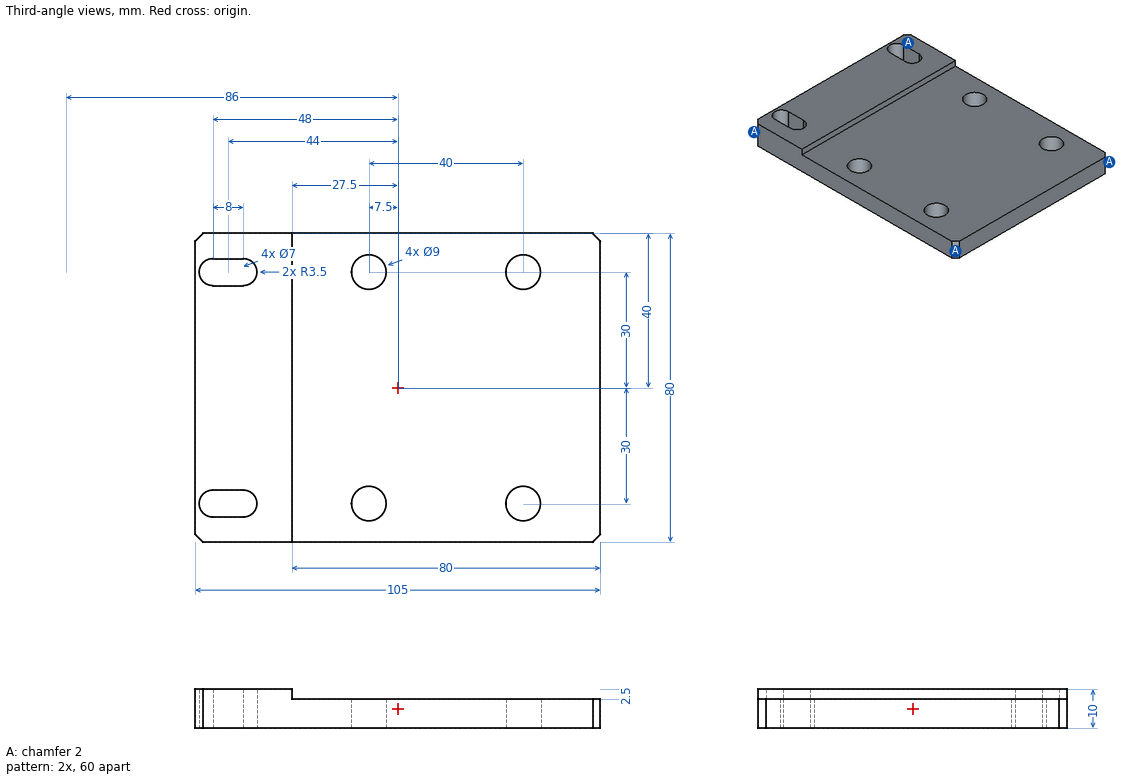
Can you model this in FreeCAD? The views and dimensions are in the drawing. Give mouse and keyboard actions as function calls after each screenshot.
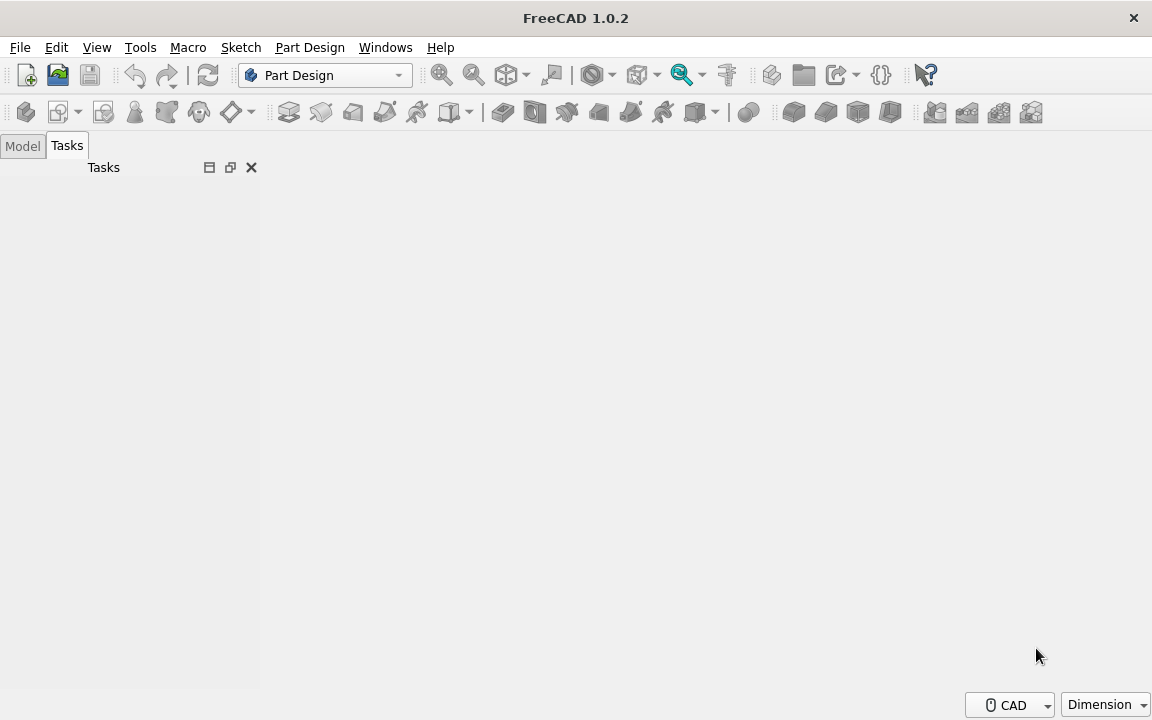
click(26, 76)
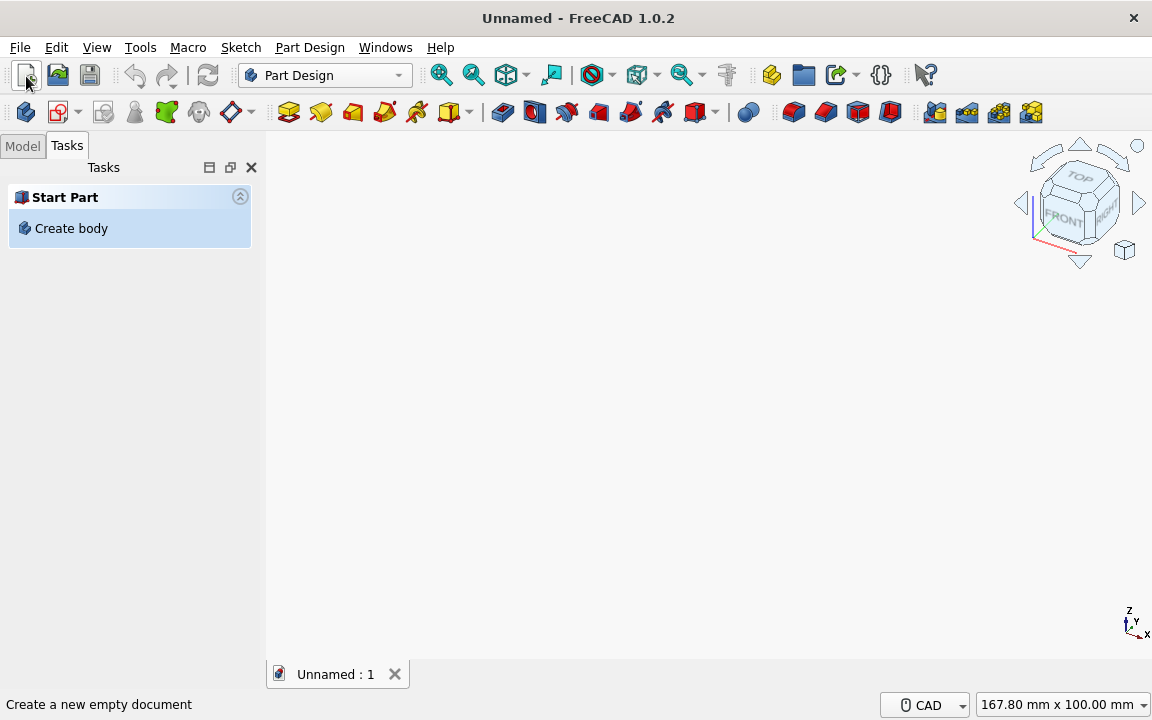
click(58, 112)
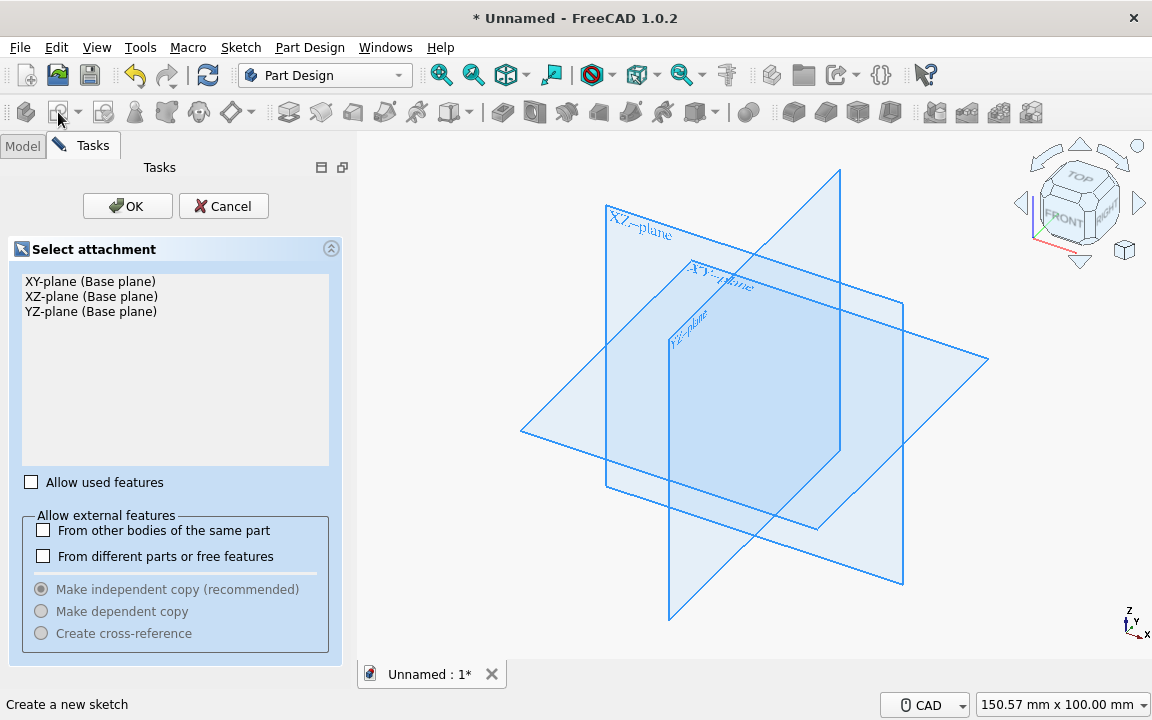
click(82, 282)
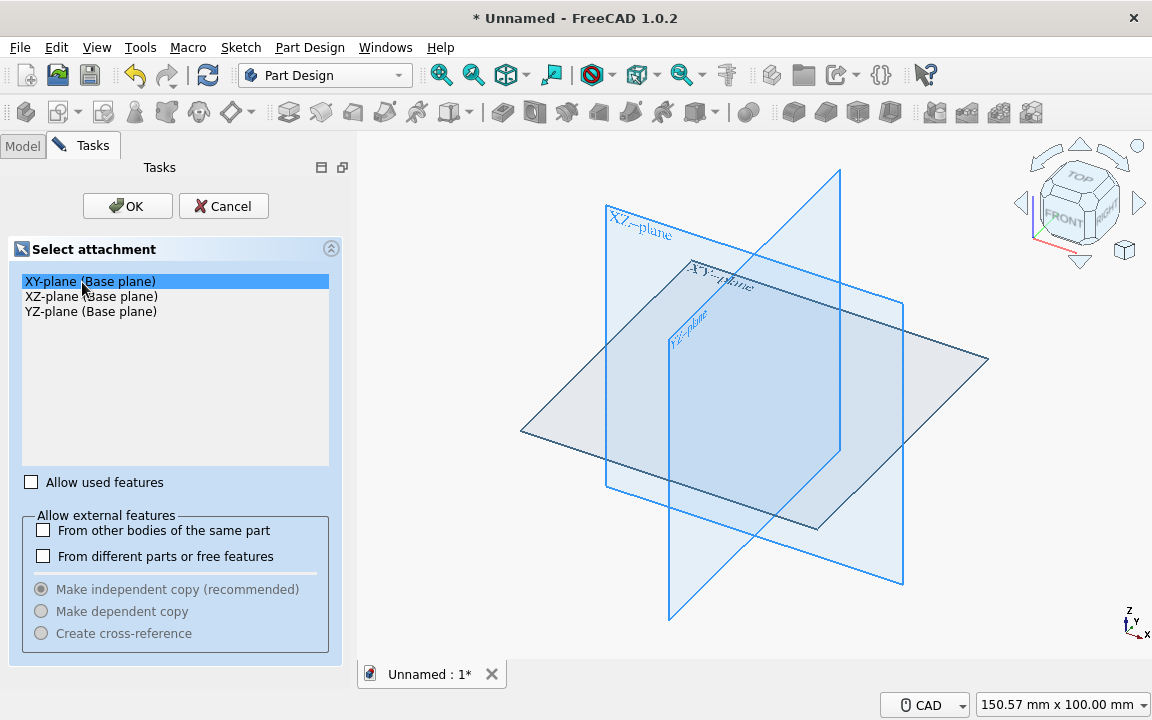
click(128, 206)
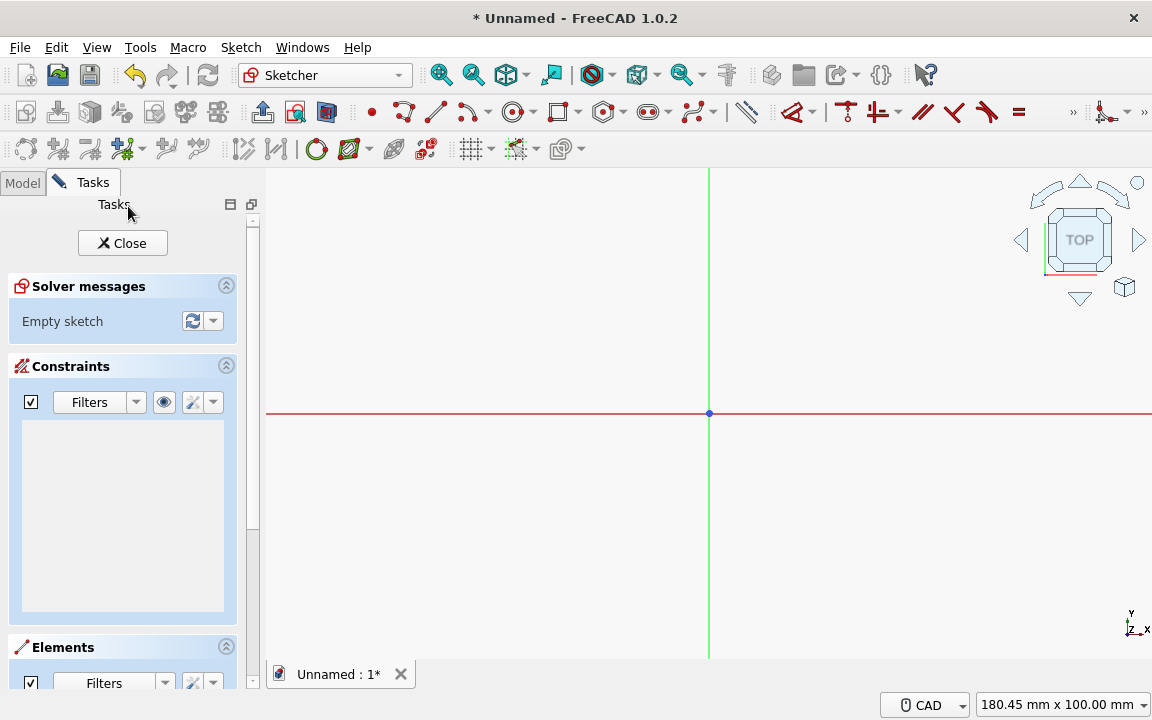
scroll(331, 413, down, 1)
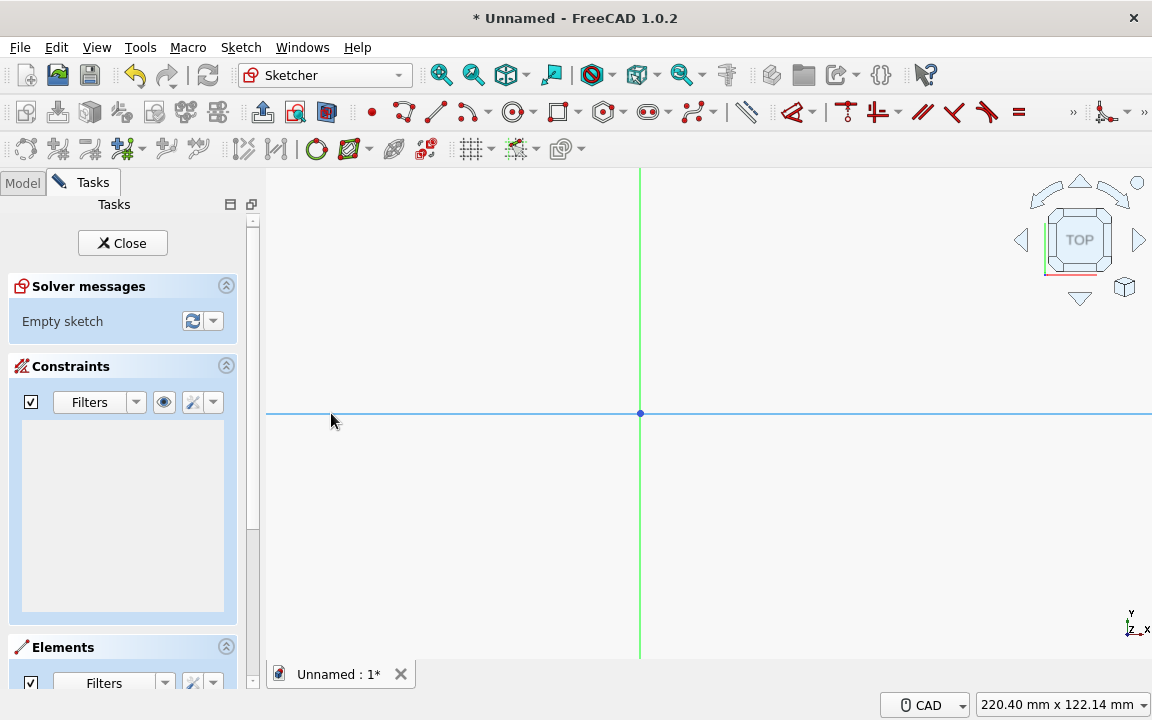
key(g)
key(v)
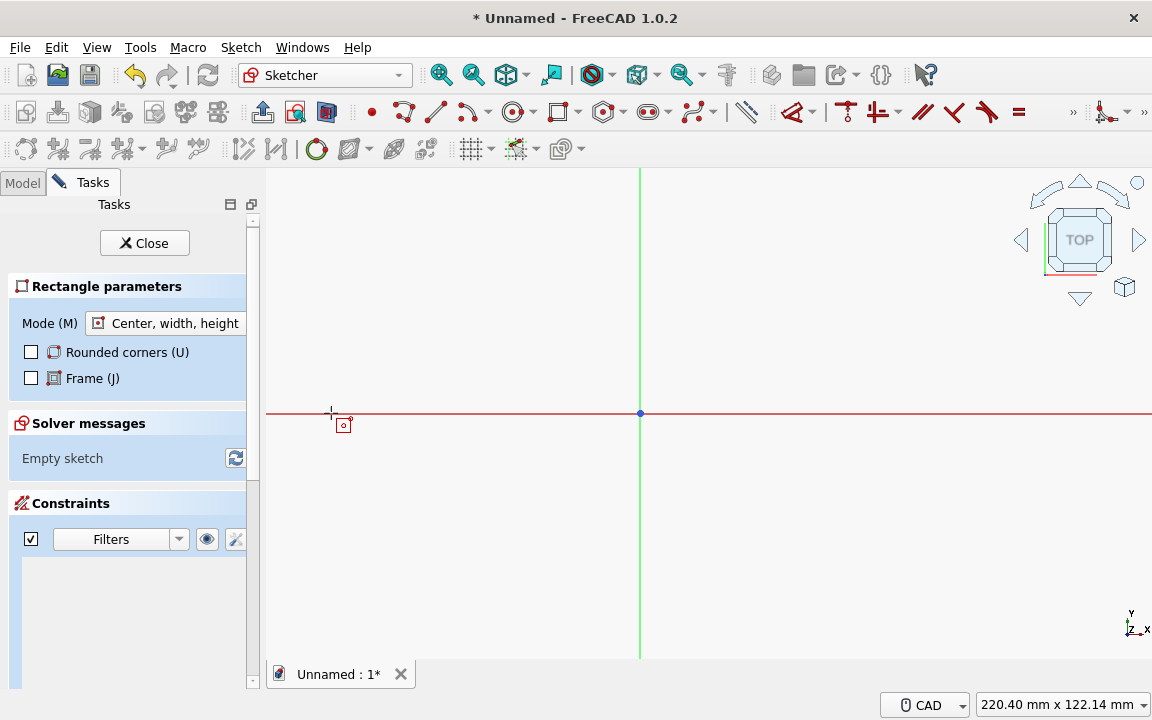
click(640, 414)
click(852, 253)
key(Escape)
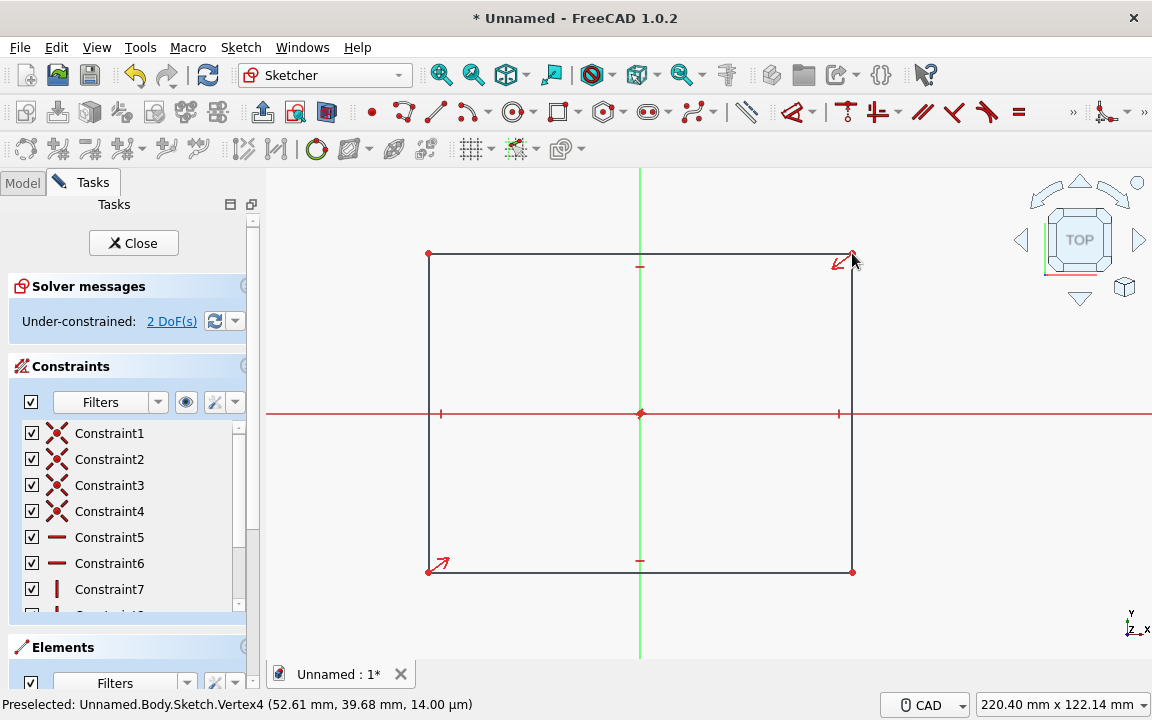
click(852, 477)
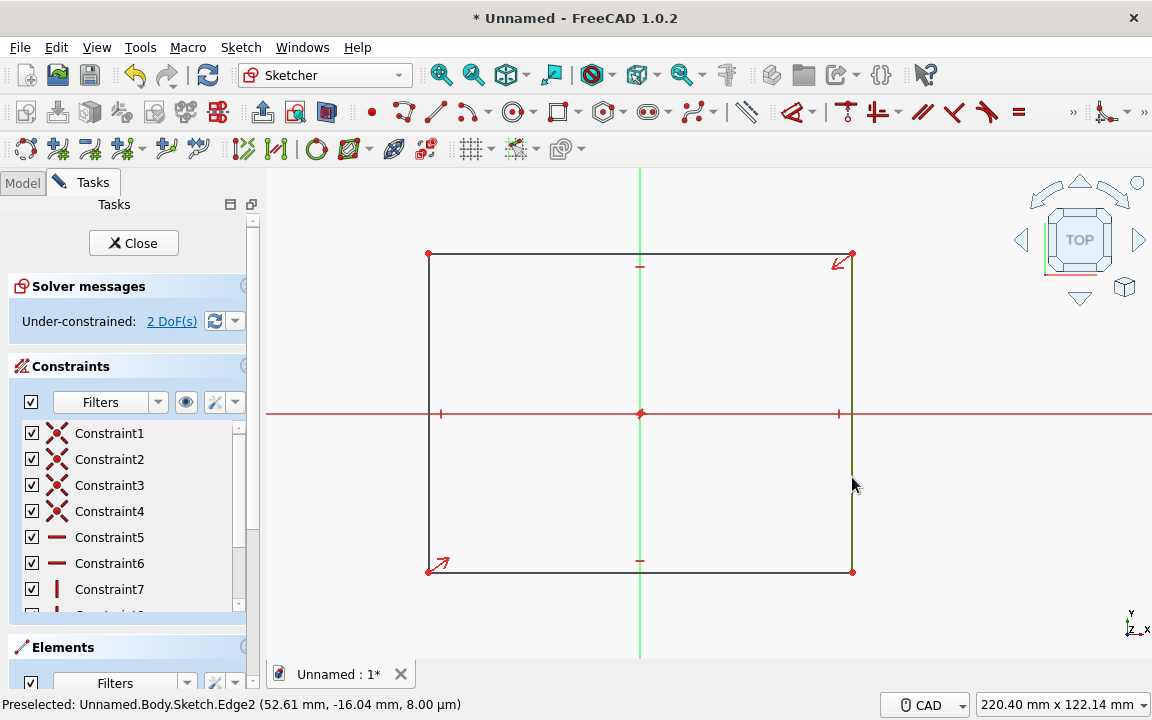
key(i)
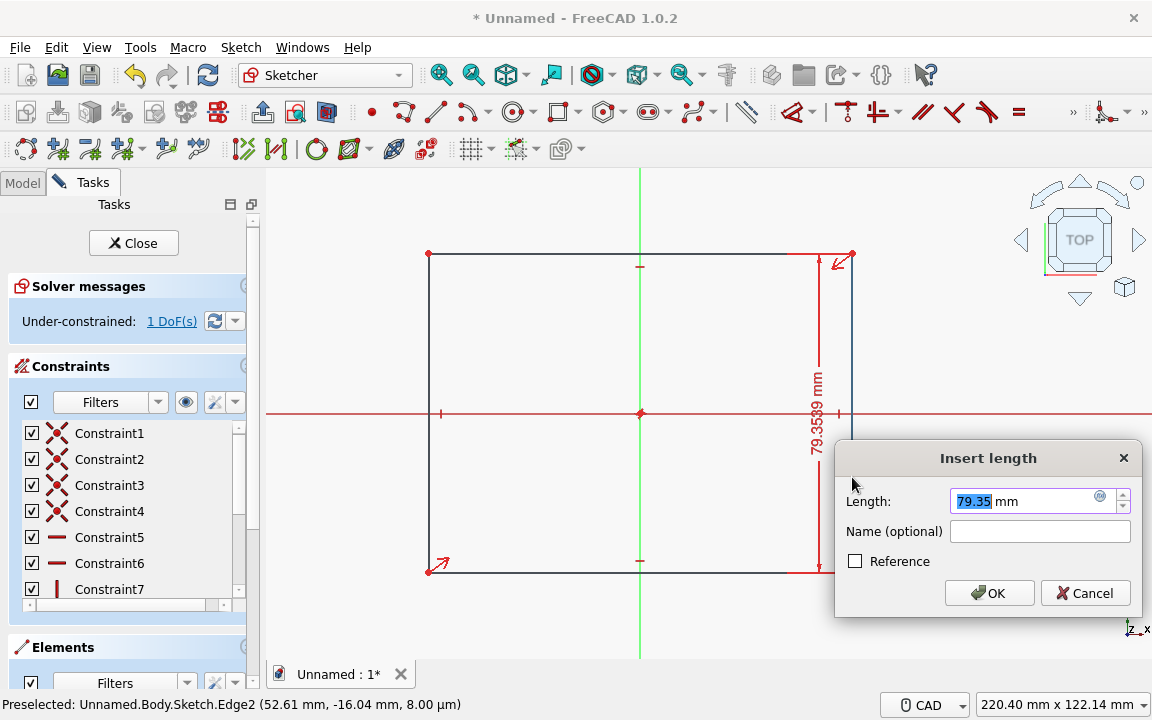
text(80)
key(Return)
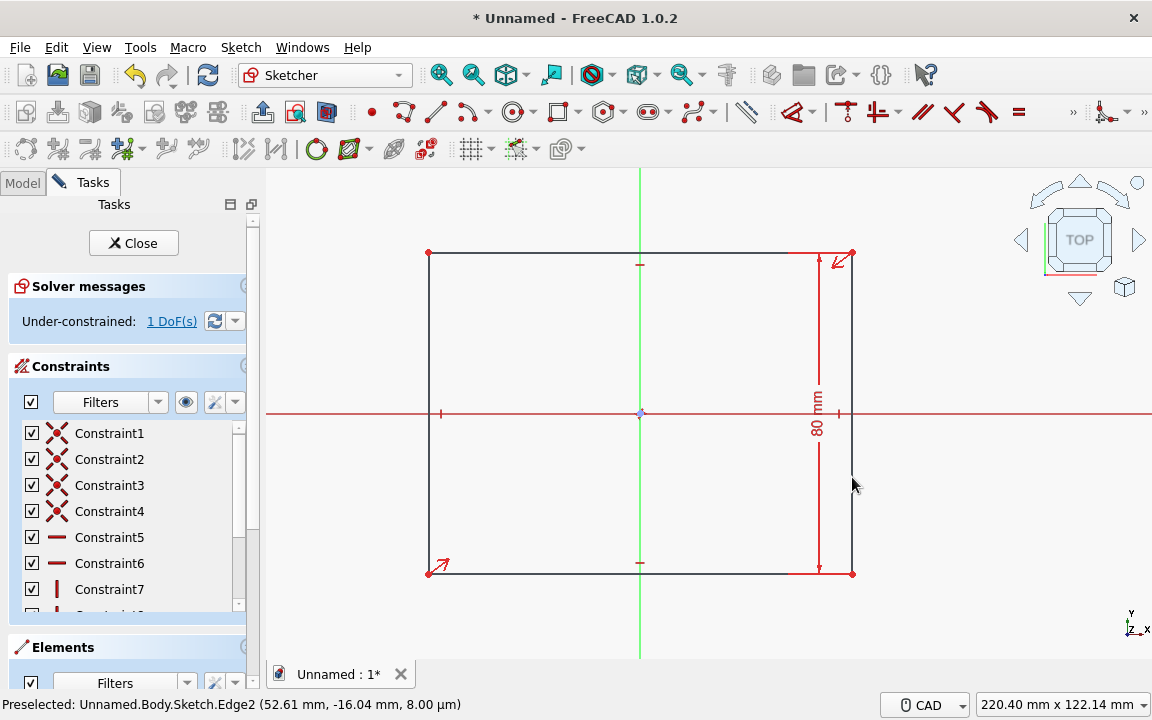
click(556, 574)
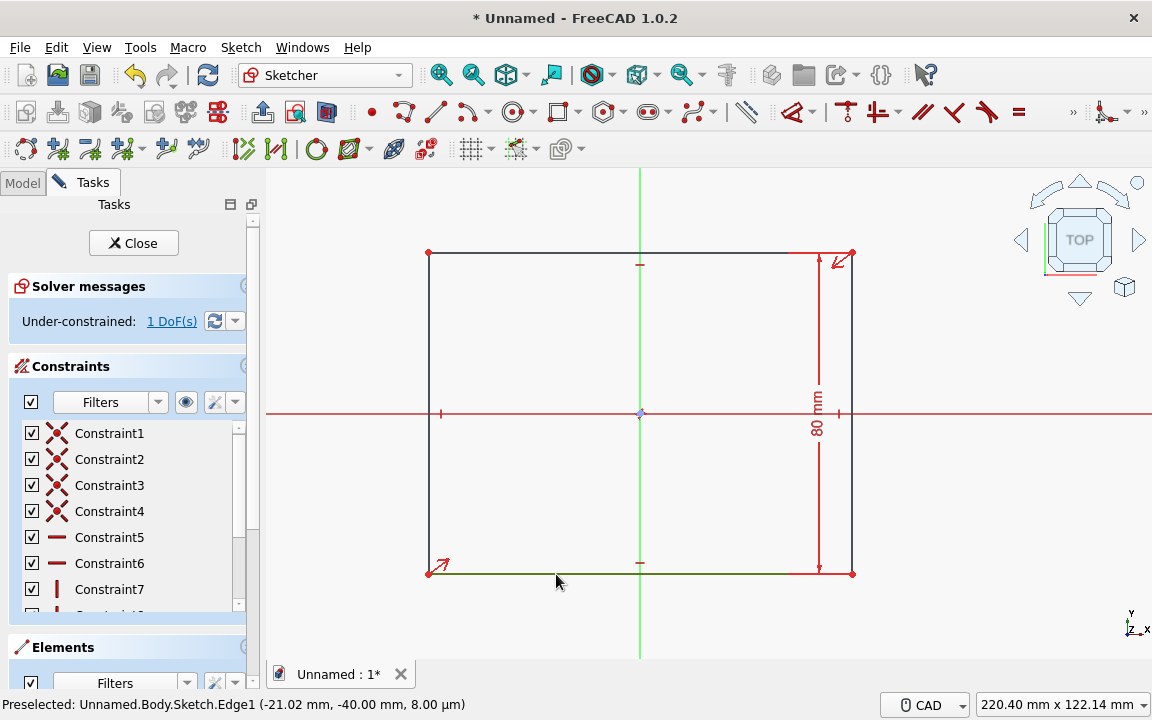
key(l)